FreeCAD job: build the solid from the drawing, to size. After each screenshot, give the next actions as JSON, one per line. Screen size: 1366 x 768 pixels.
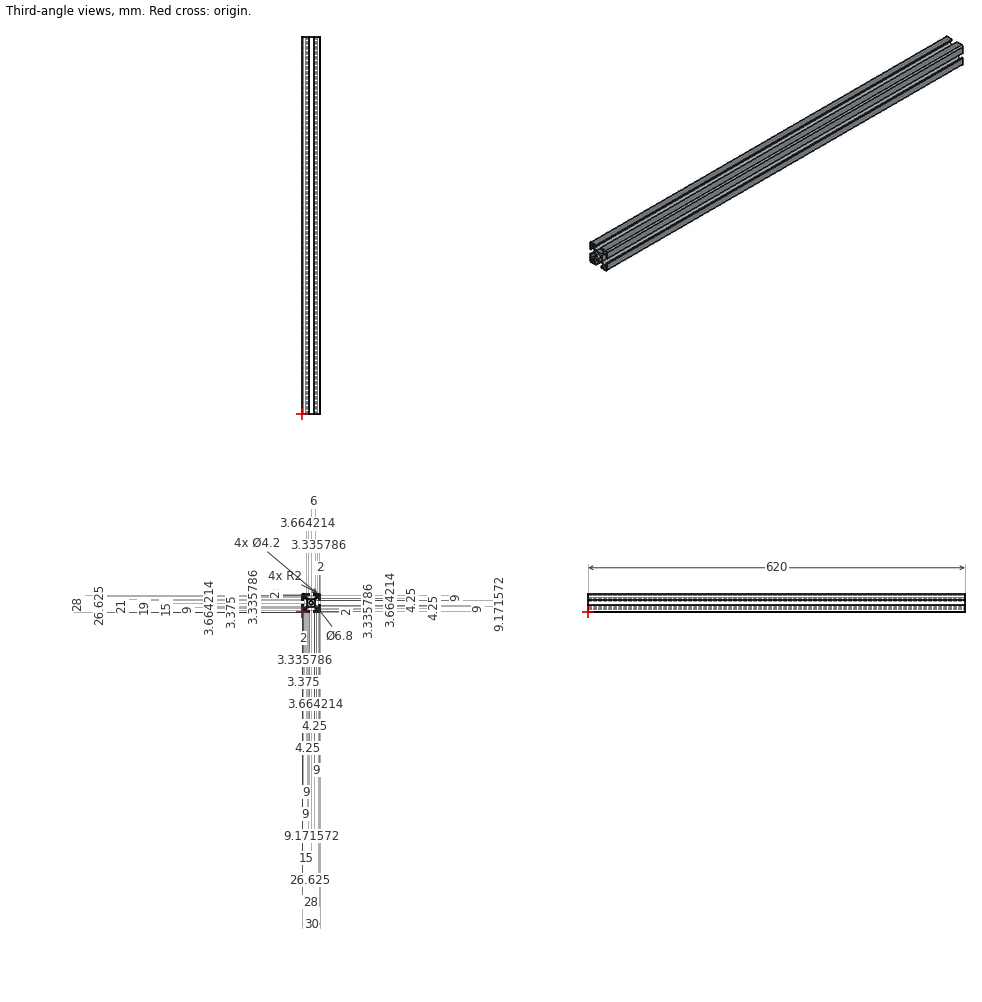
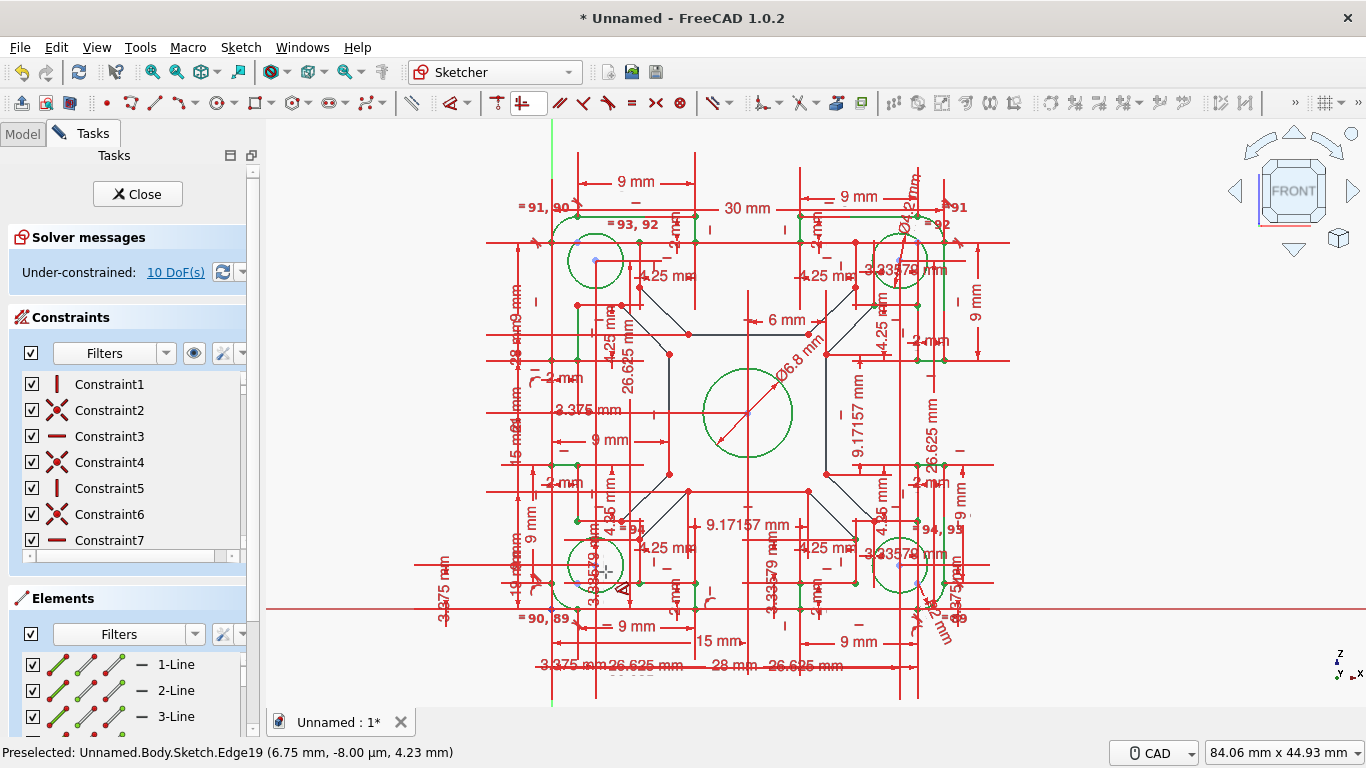
{"action": "left_click", "coordinate": [591, 521]}
{"action": "left_click", "coordinate": [599, 463]}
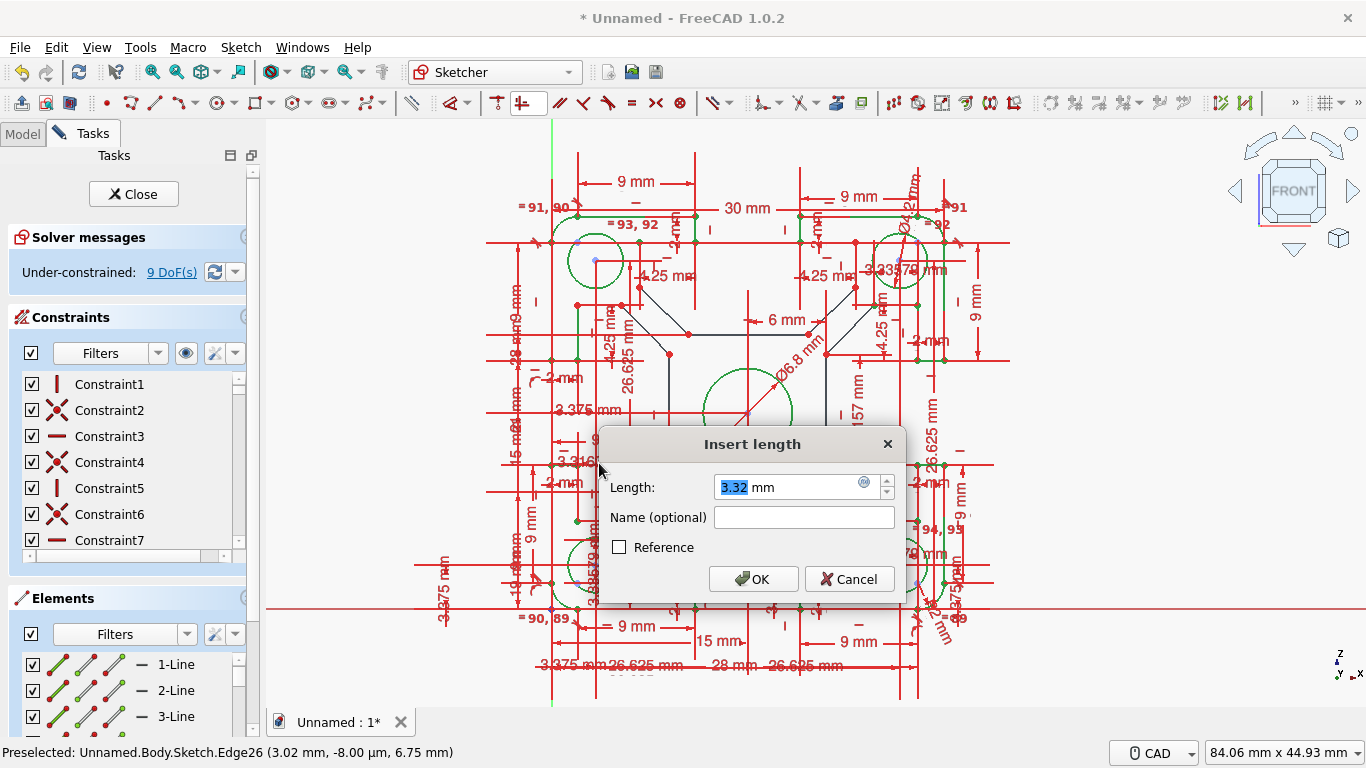
{"action": "type", "text": "3.335786"}
{"action": "key", "text": "Return"}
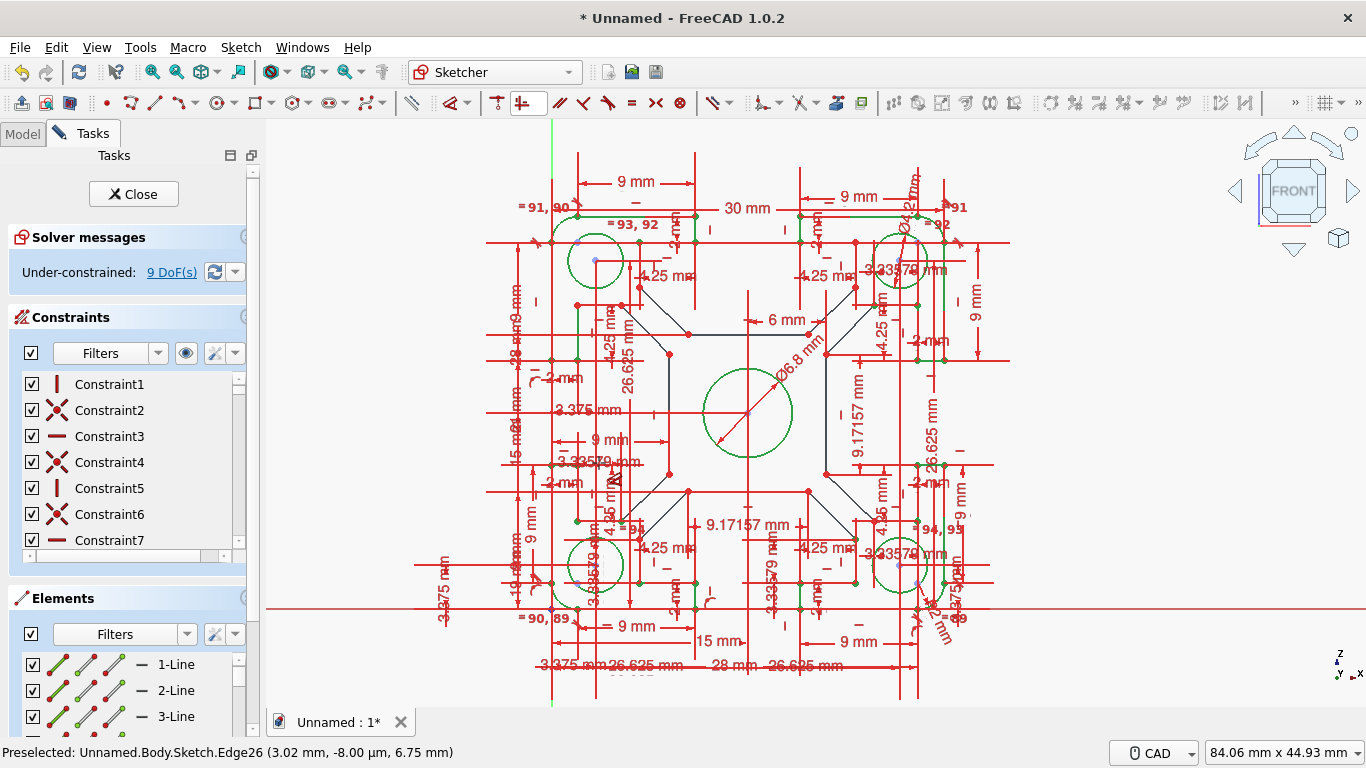
{"action": "left_click", "coordinate": [669, 439]}
{"action": "left_click", "coordinate": [635, 387]}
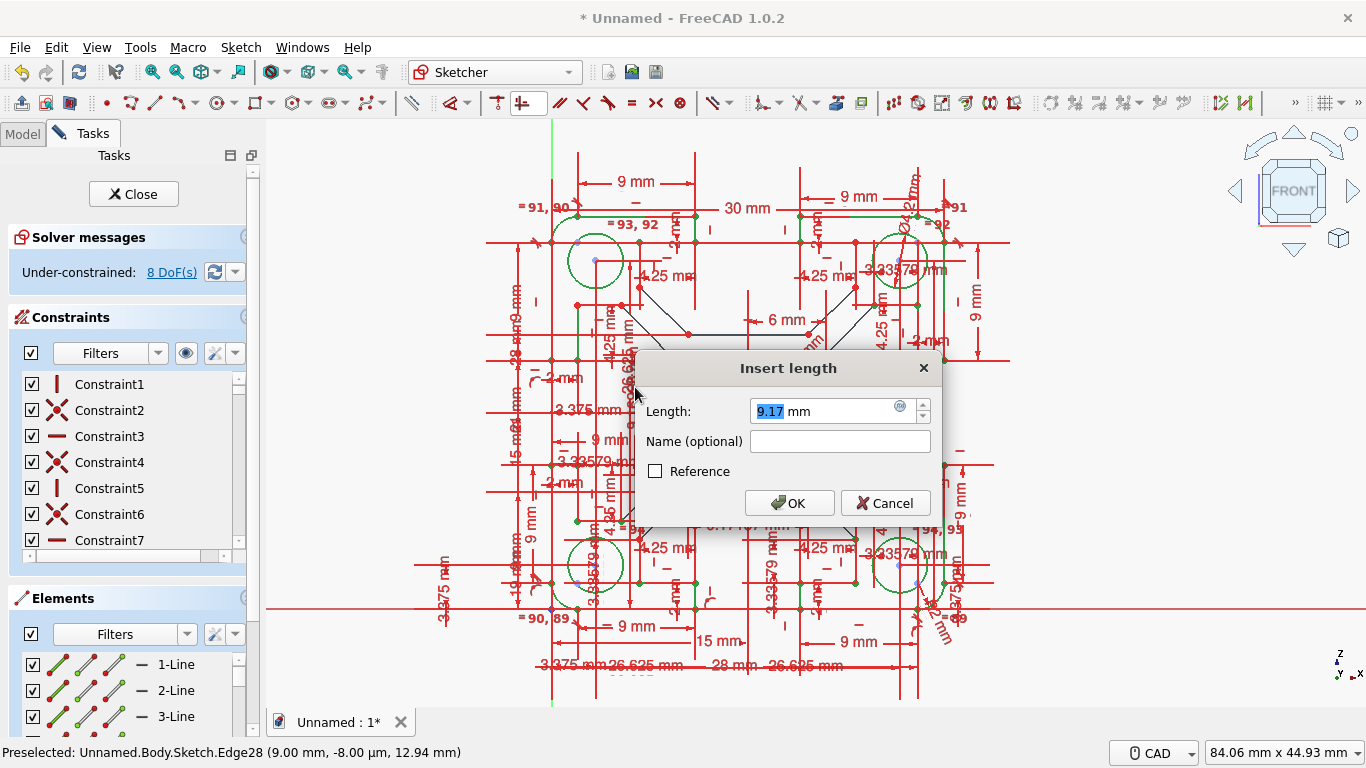
{"action": "type", "text": "9.171572"}
{"action": "key", "text": "Return"}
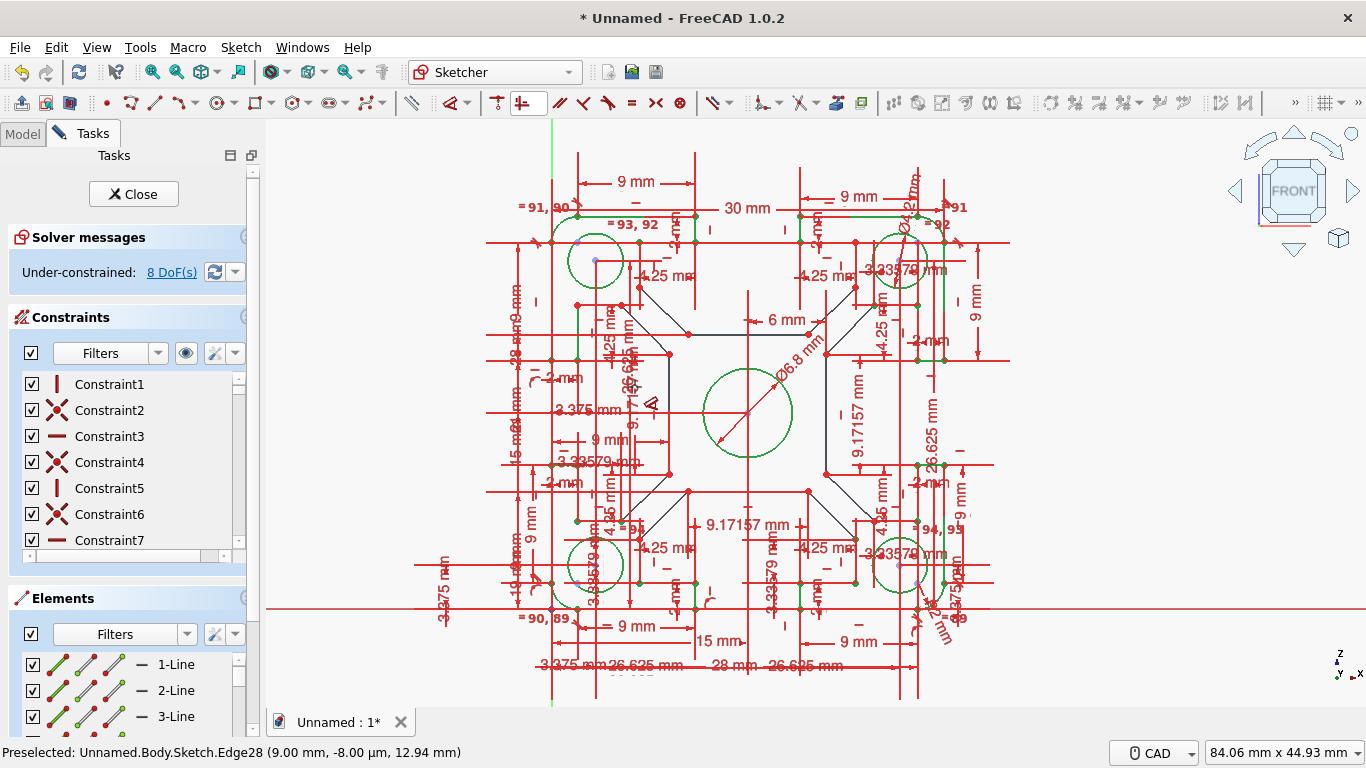
{"action": "left_click", "coordinate": [608, 305]}
{"action": "left_click", "coordinate": [589, 271]}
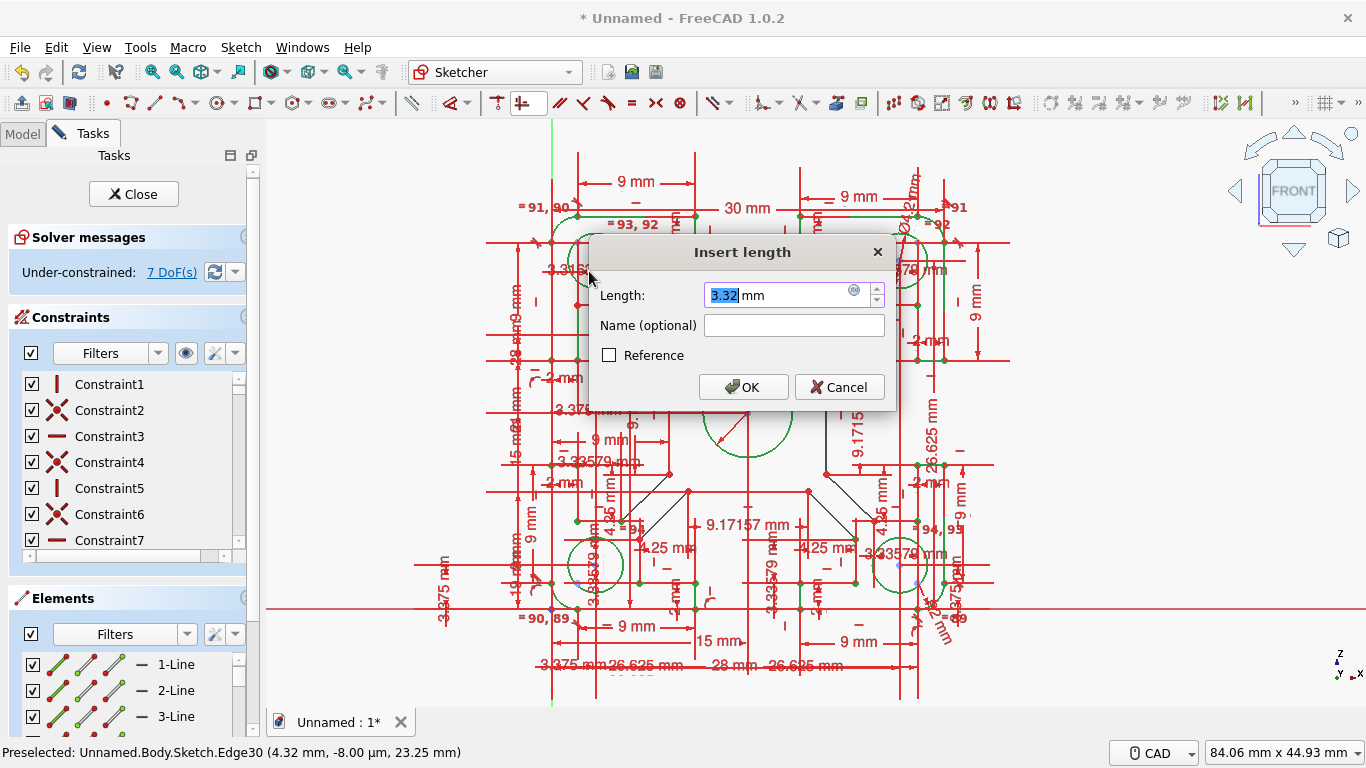
{"action": "type", "text": "3.335786"}
{"action": "key", "text": "Return"}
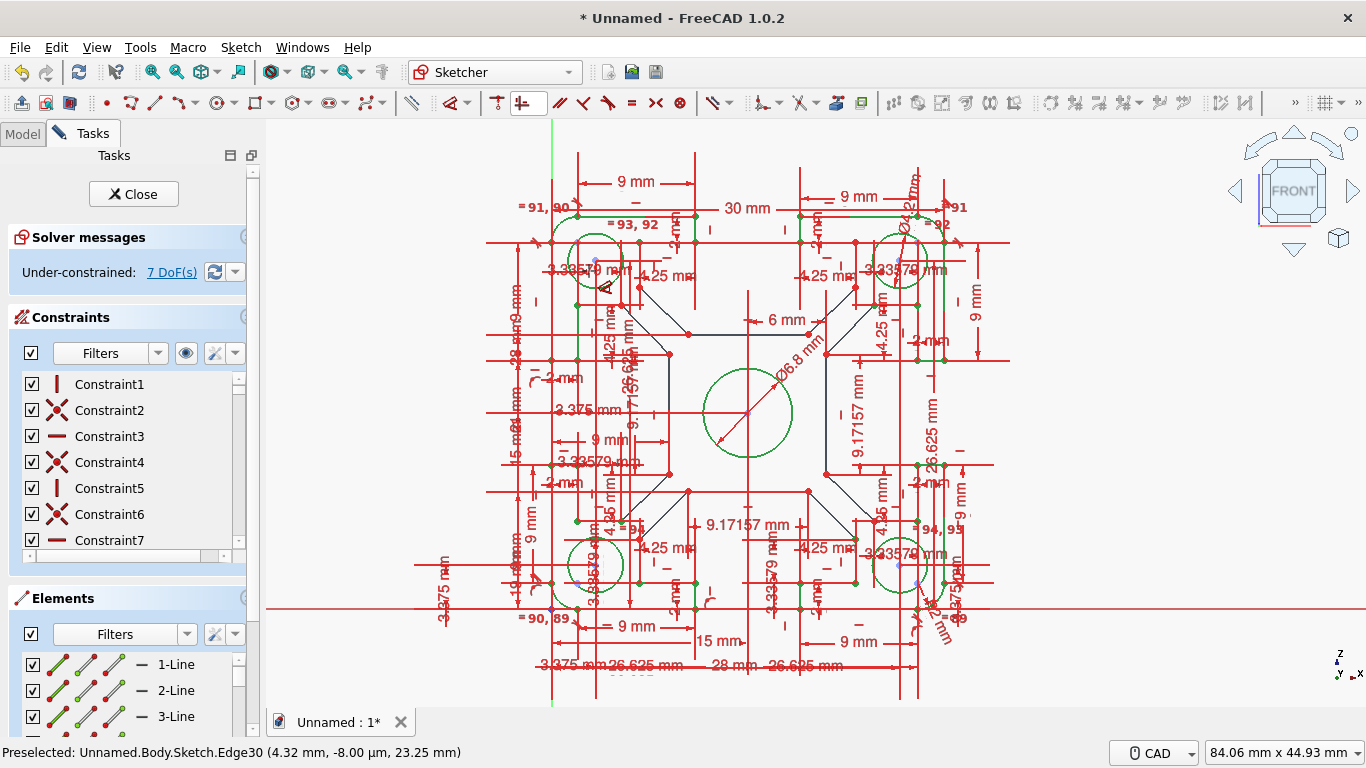
{"action": "left_click", "coordinate": [640, 256]}
{"action": "left_click", "coordinate": [722, 255]}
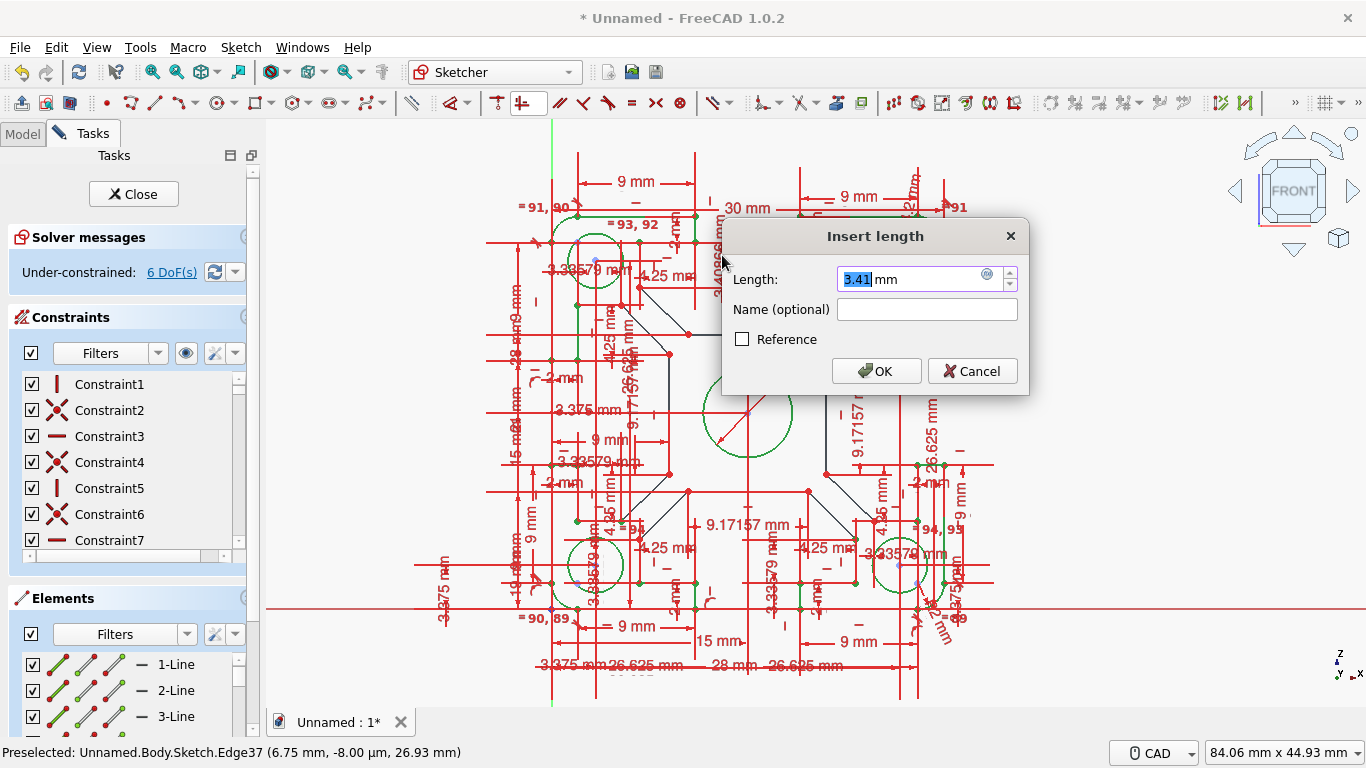
{"action": "type", "text": "3.335786"}
{"action": "key", "text": "Return"}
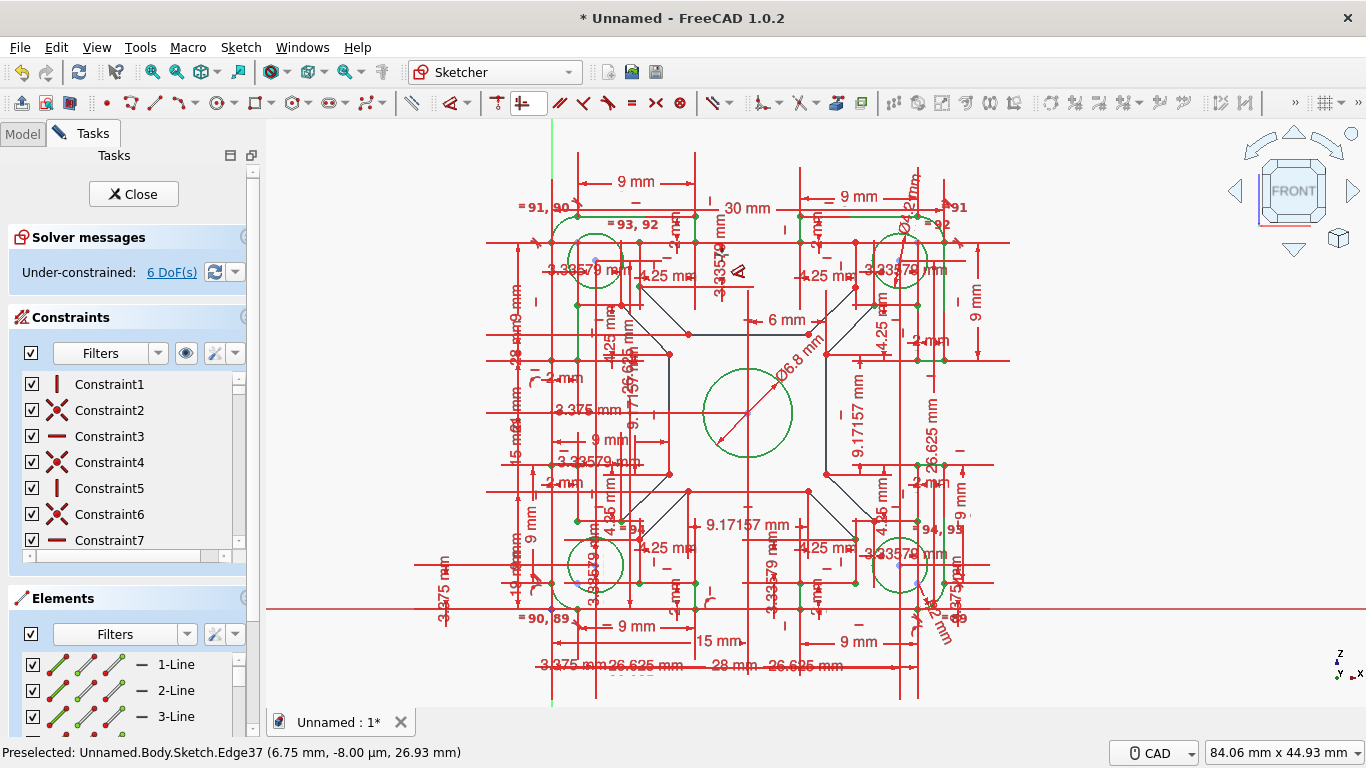
{"action": "left_click", "coordinate": [724, 335]}
{"action": "left_click", "coordinate": [748, 301]}